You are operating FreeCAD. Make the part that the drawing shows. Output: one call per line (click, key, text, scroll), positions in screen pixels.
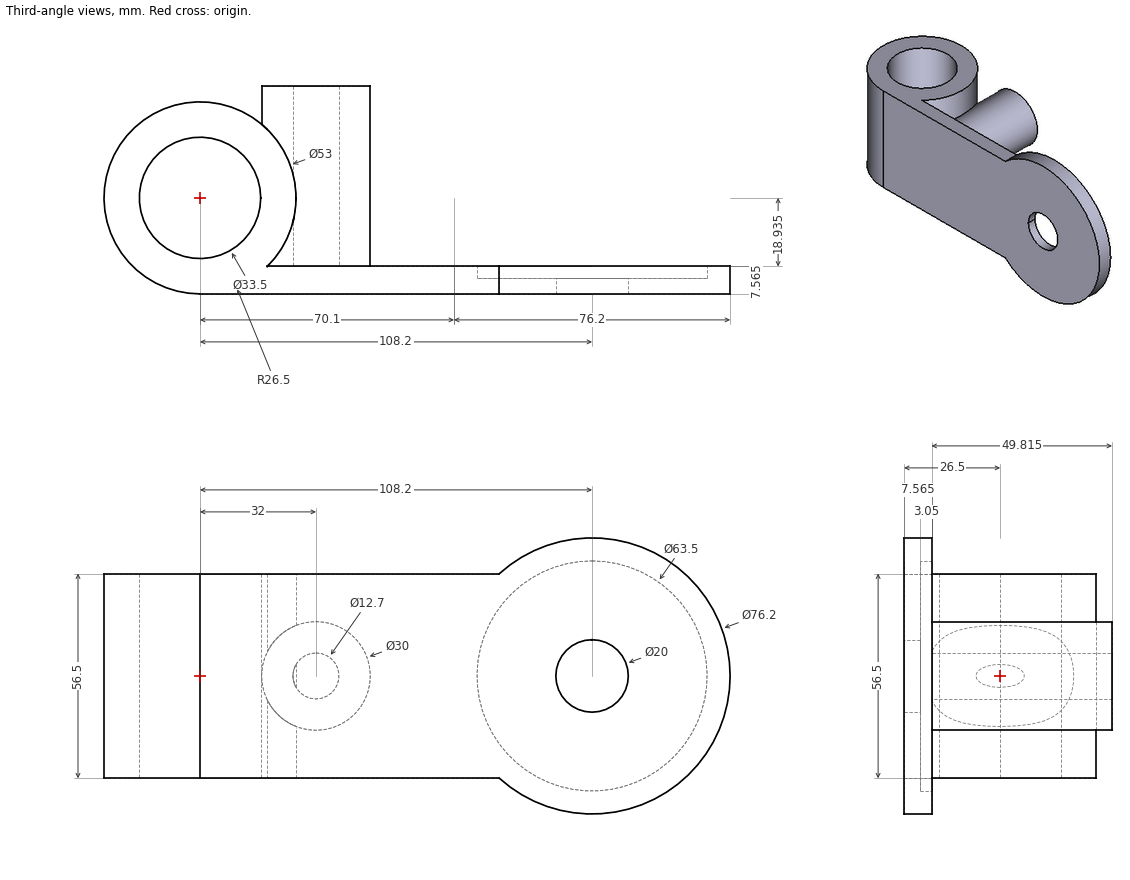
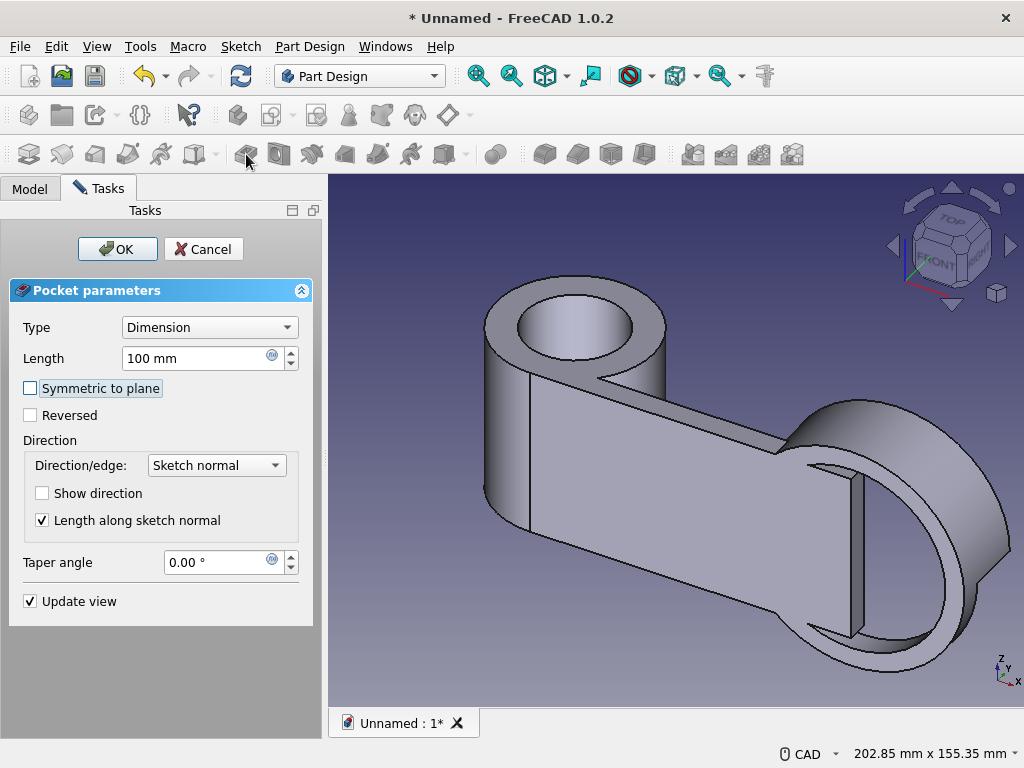
click(31, 388)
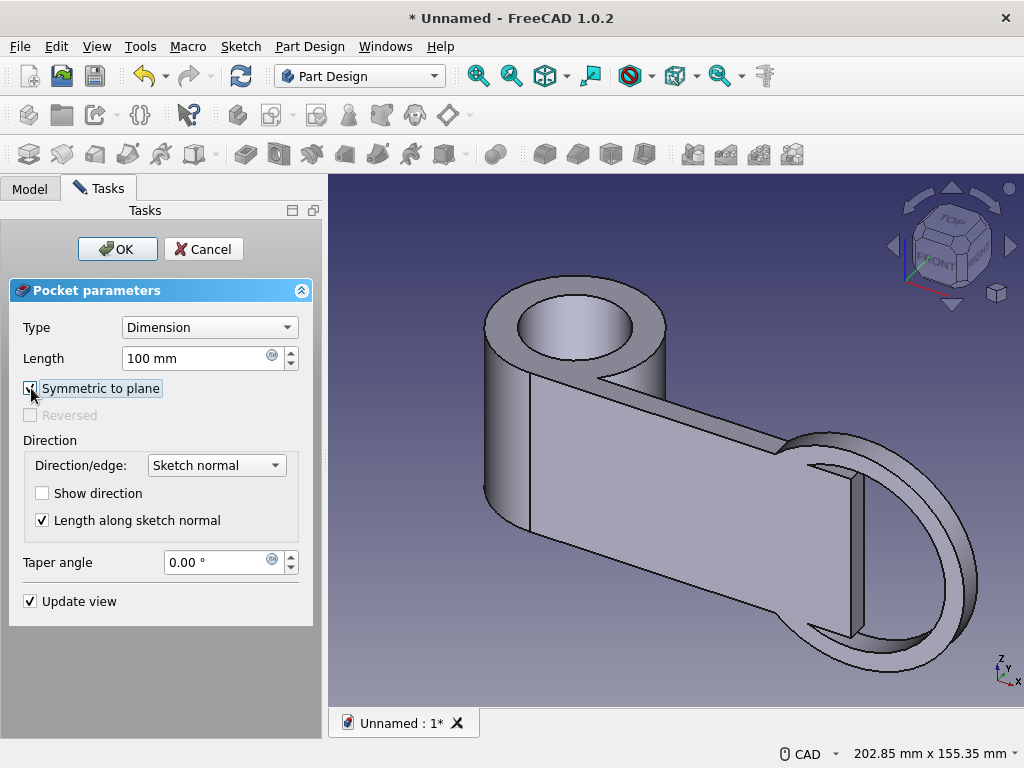
click(118, 249)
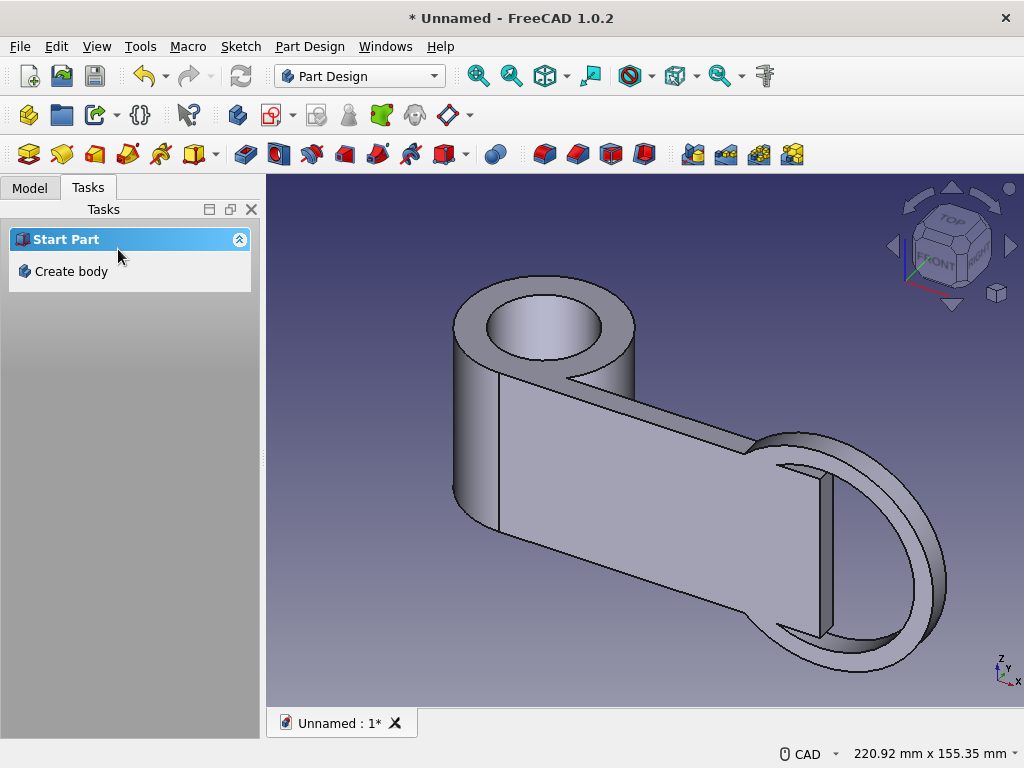
key(4)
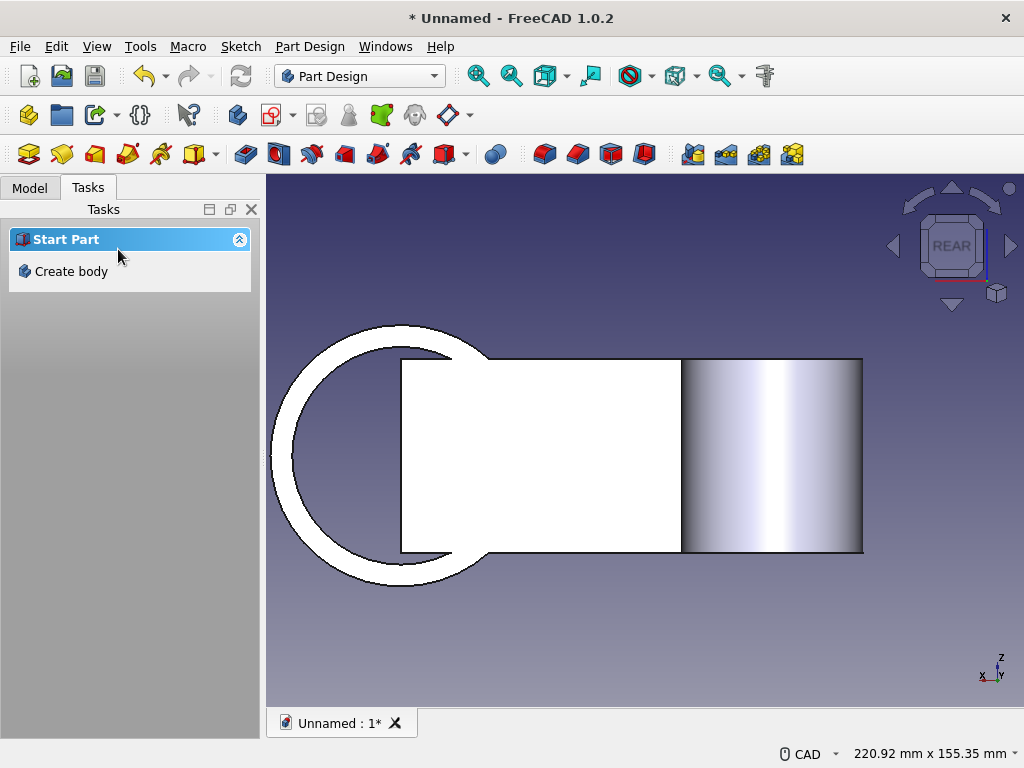
click(552, 455)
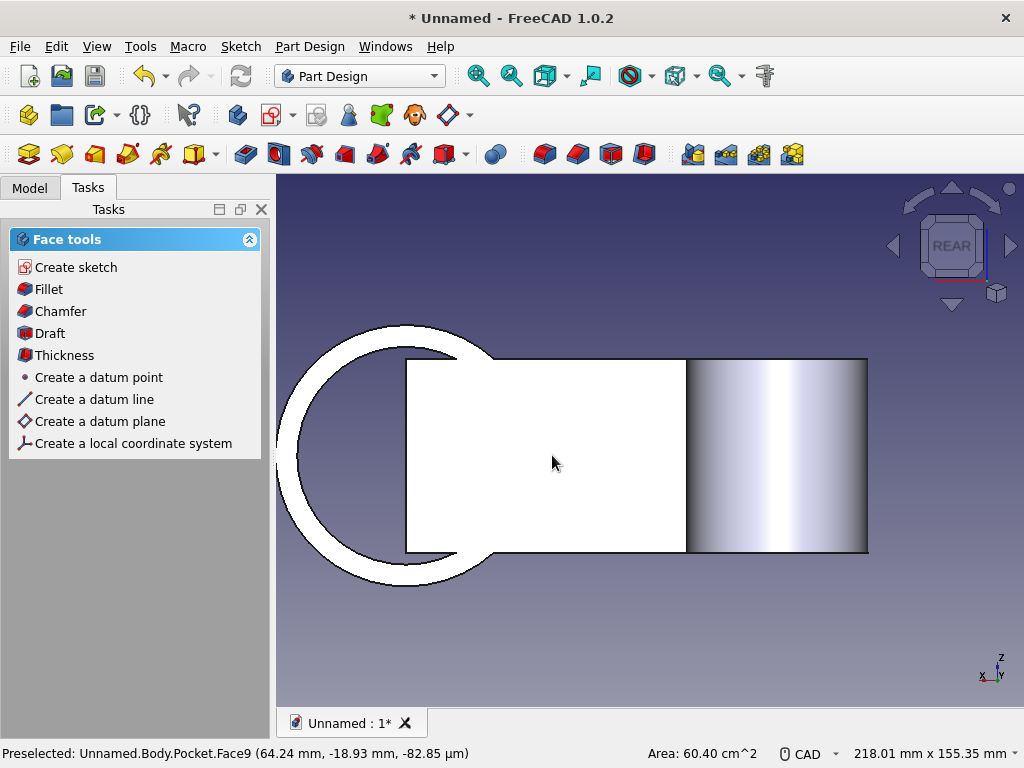
click(270, 116)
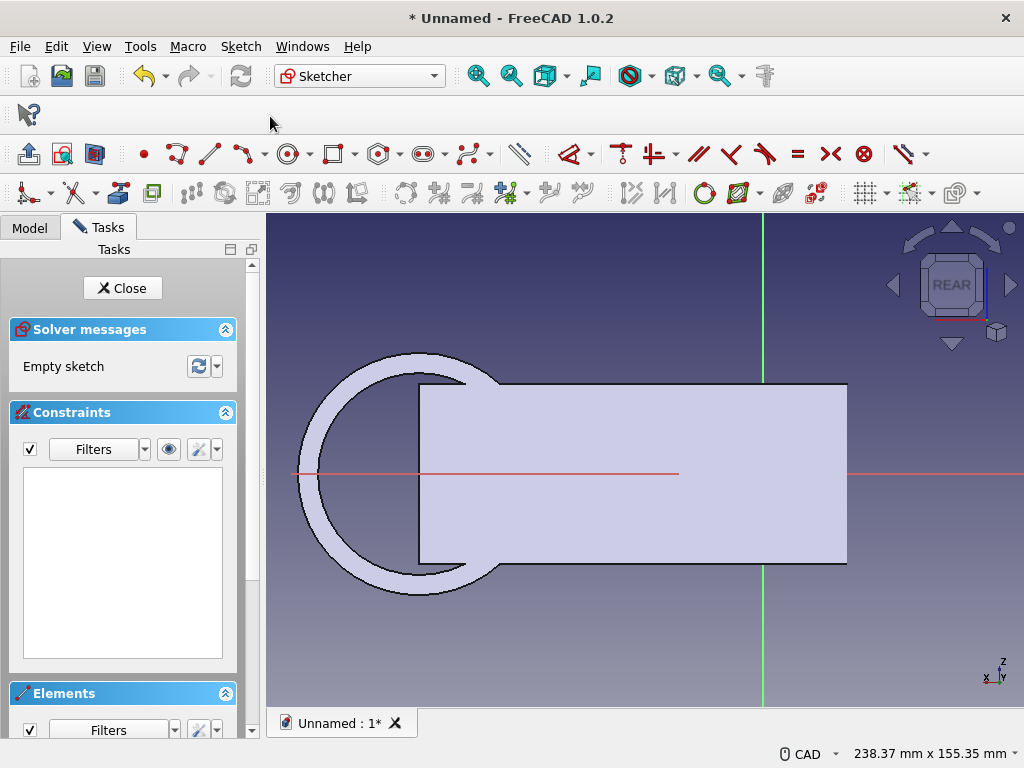
click(95, 154)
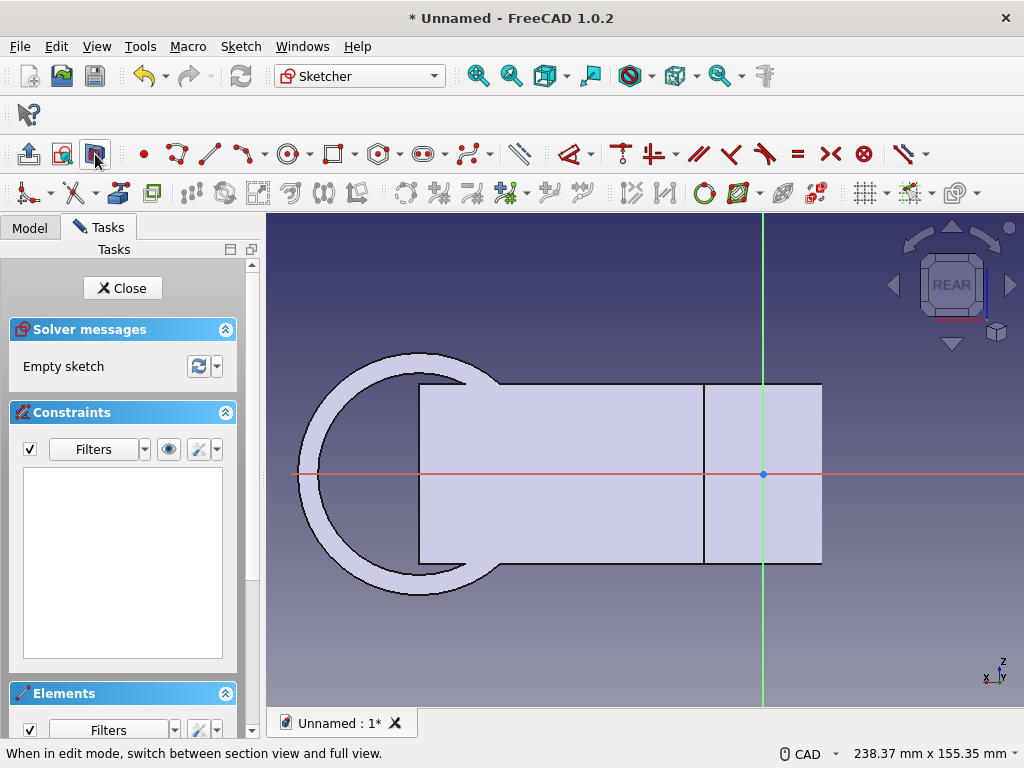
scroll(739, 396, down, 1)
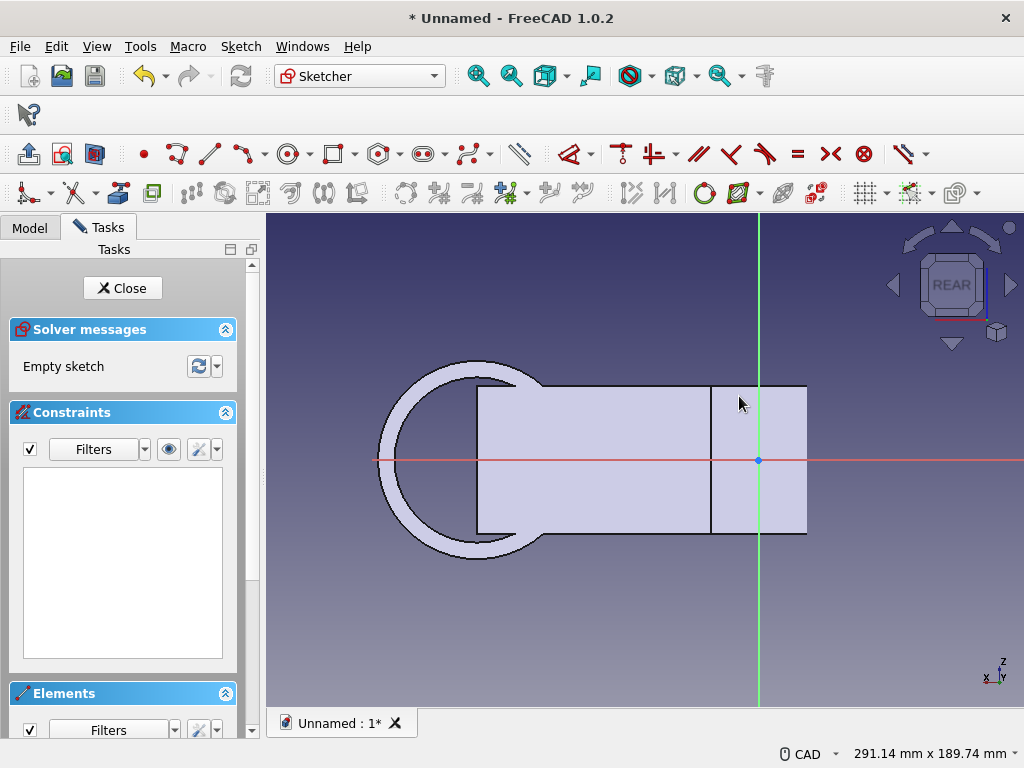
click(288, 154)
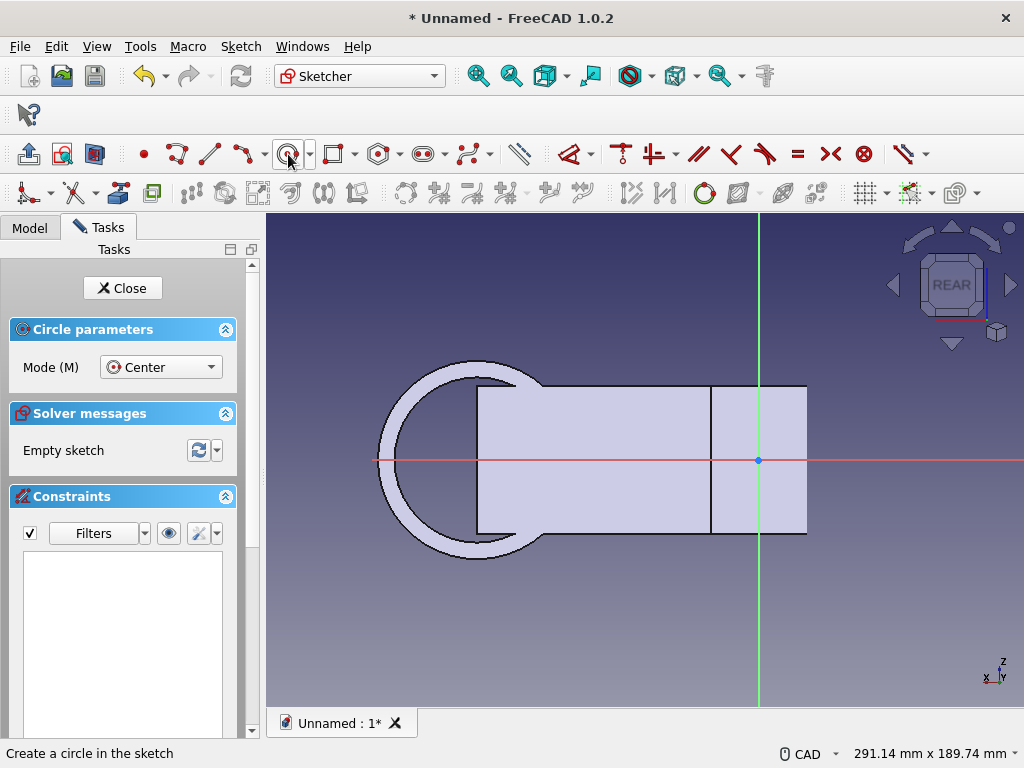
click(477, 460)
move(536, 402)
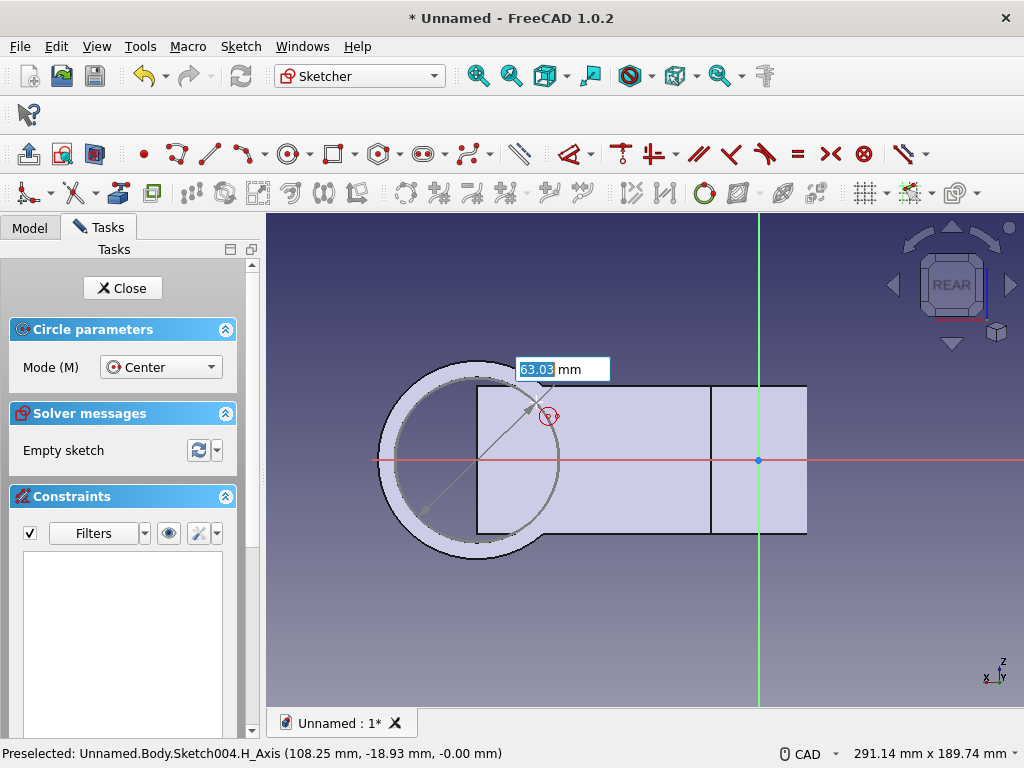
text(63.5)
key(Return)
key(Escape)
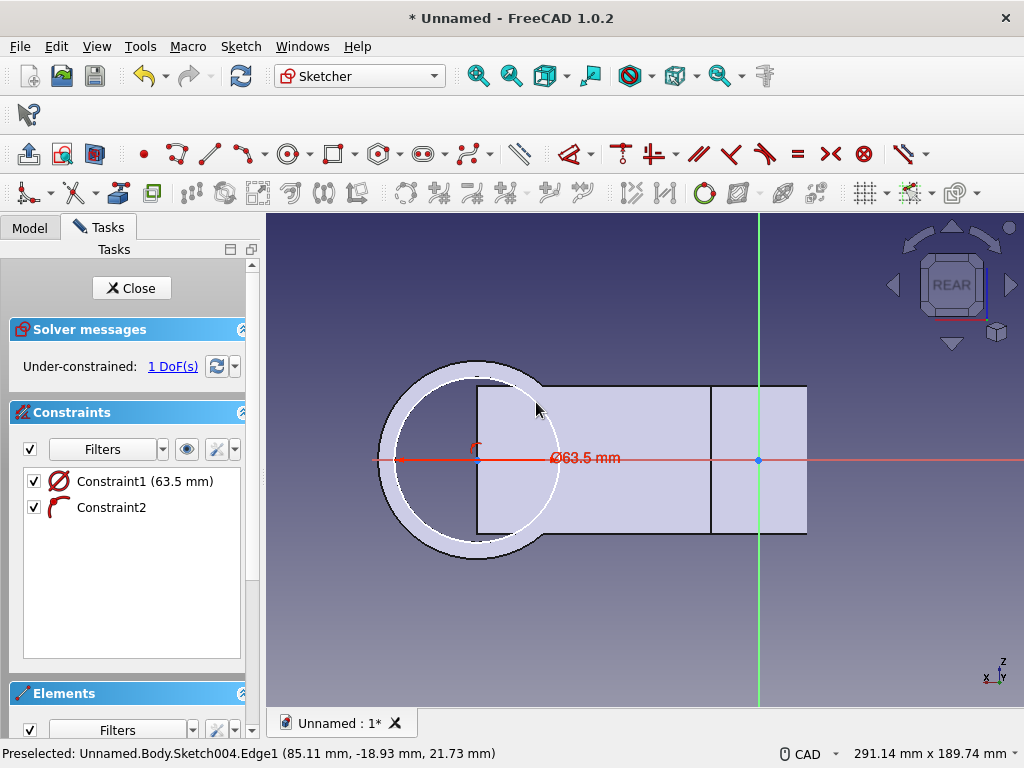
key(d)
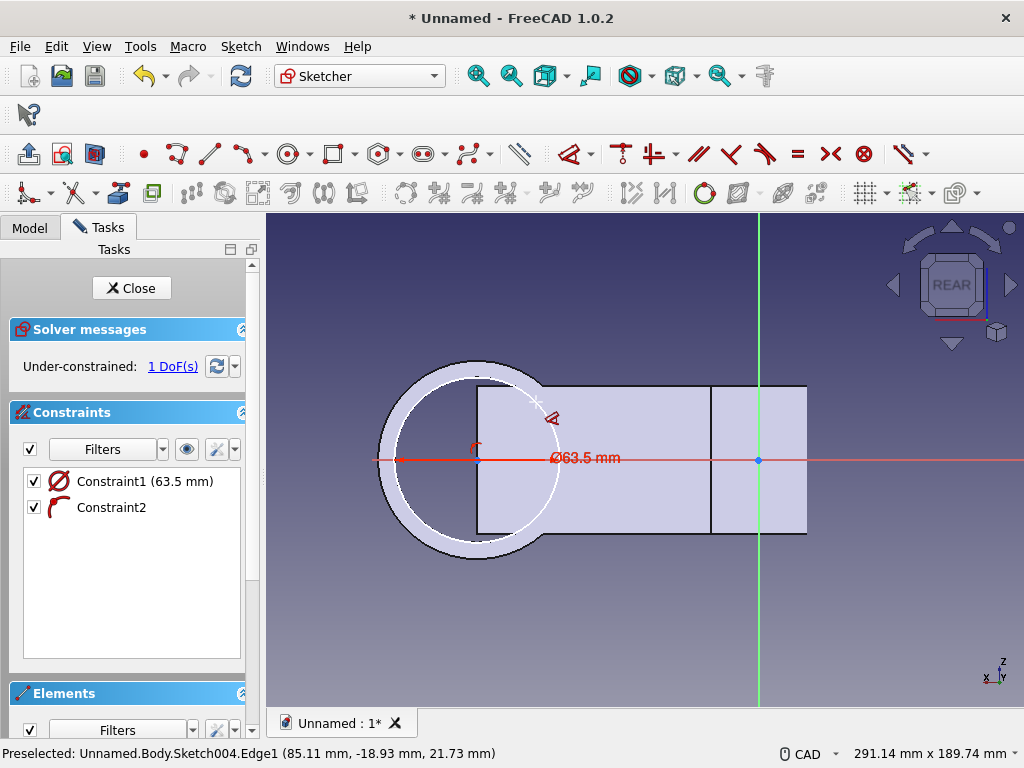
click(477, 460)
click(618, 494)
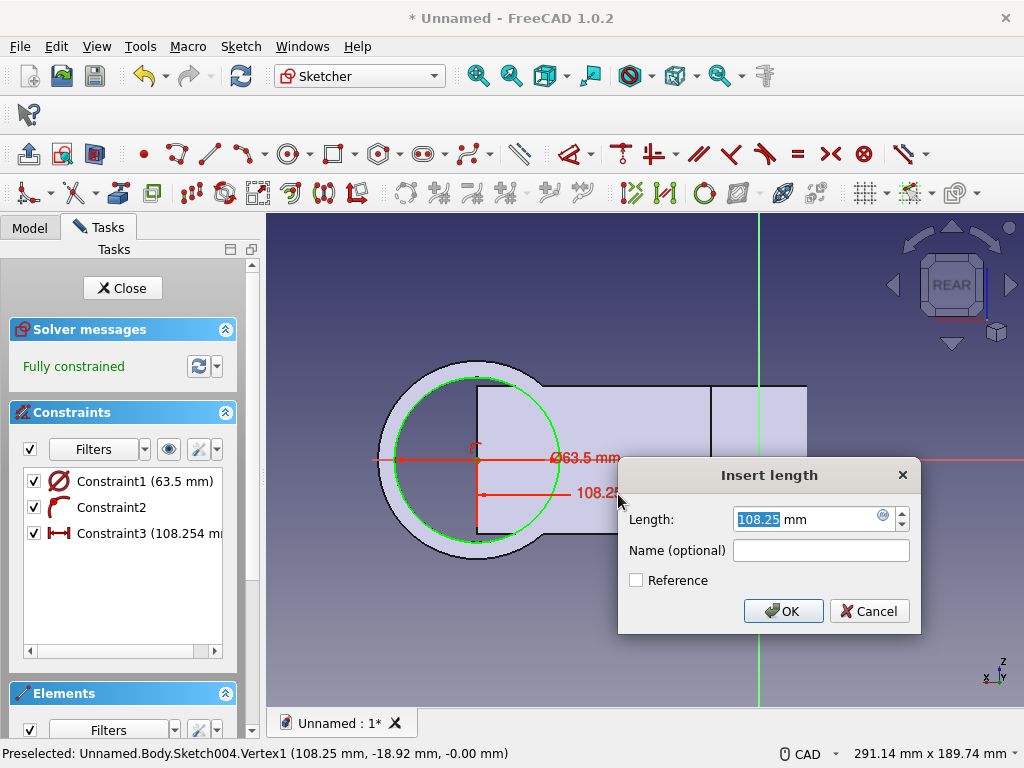
text(108.2)
key(Return)
key(Escape)